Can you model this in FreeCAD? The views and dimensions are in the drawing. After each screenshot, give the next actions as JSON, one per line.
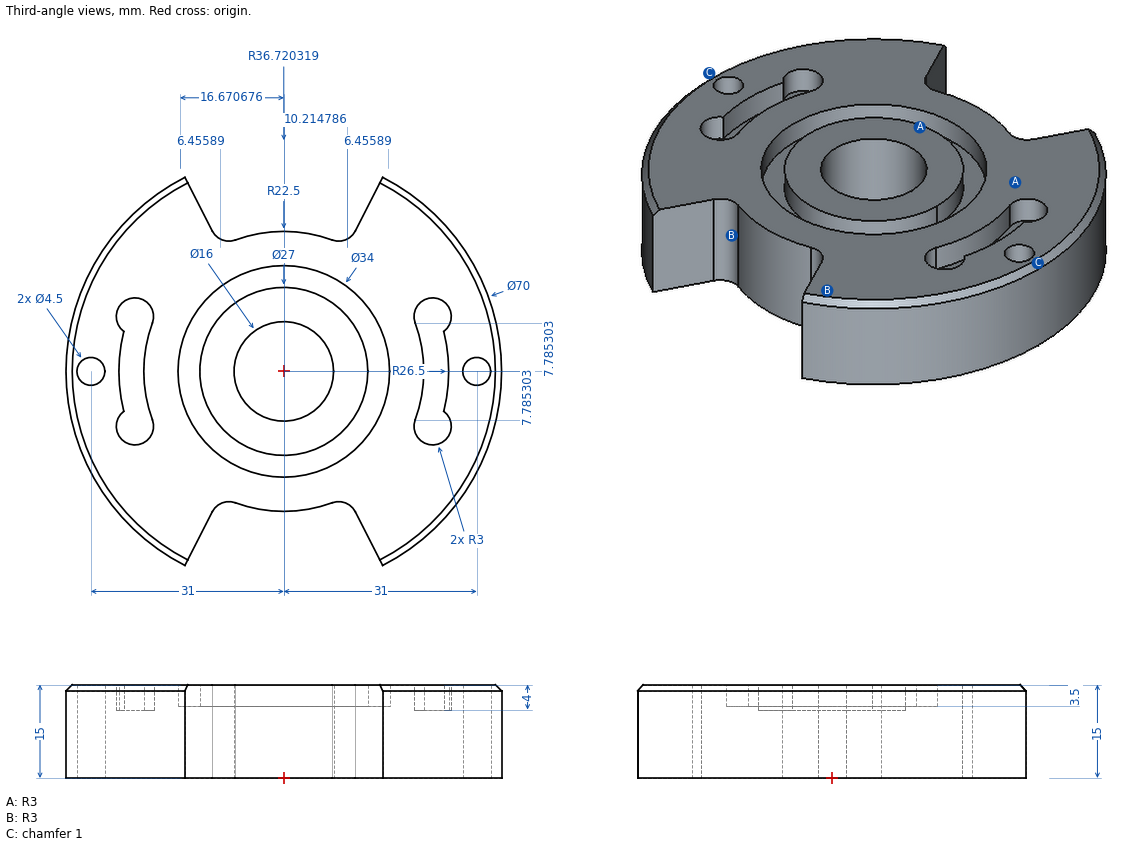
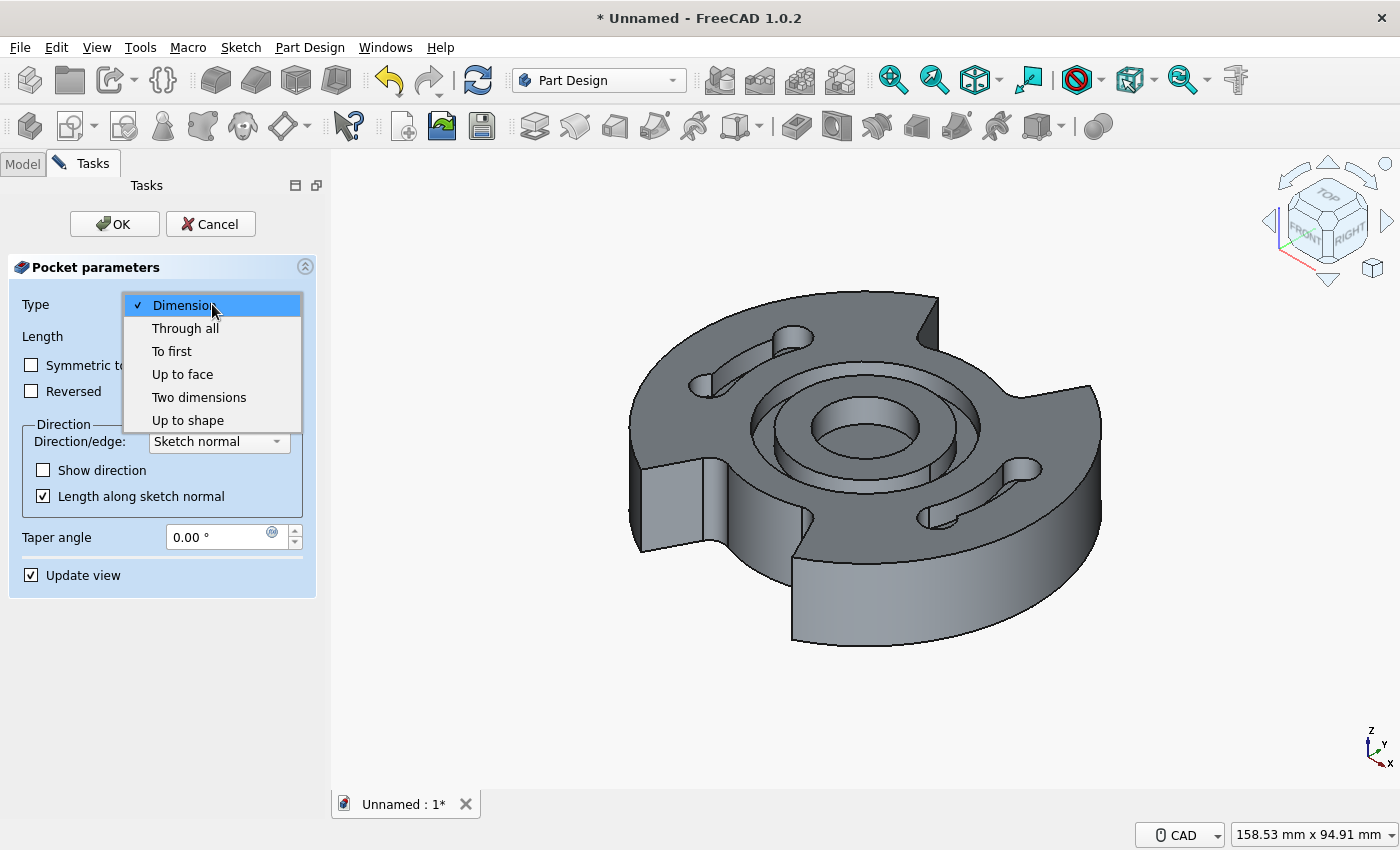
{"action": "left_click", "coordinate": [212, 328]}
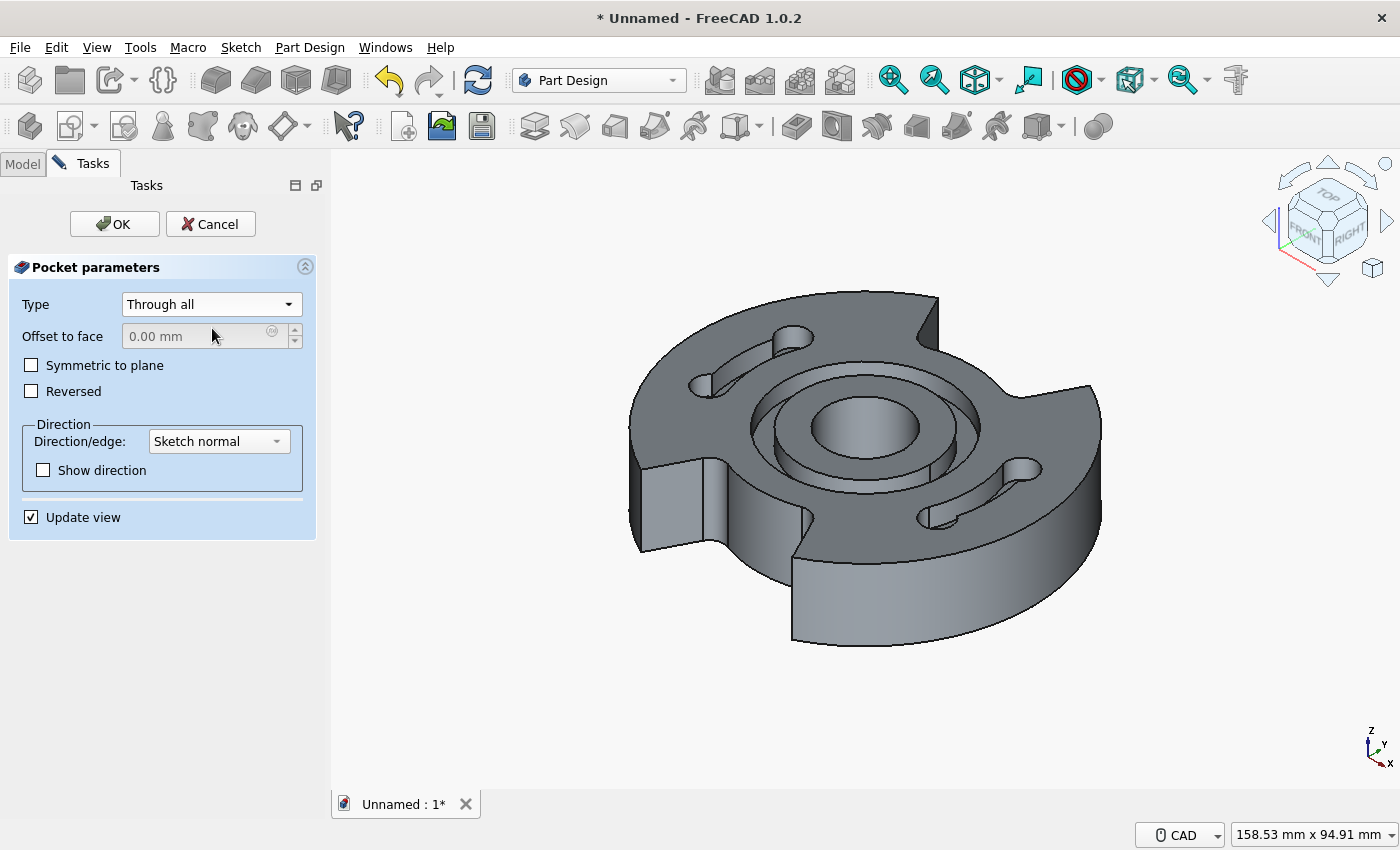
{"action": "left_click", "coordinate": [115, 224]}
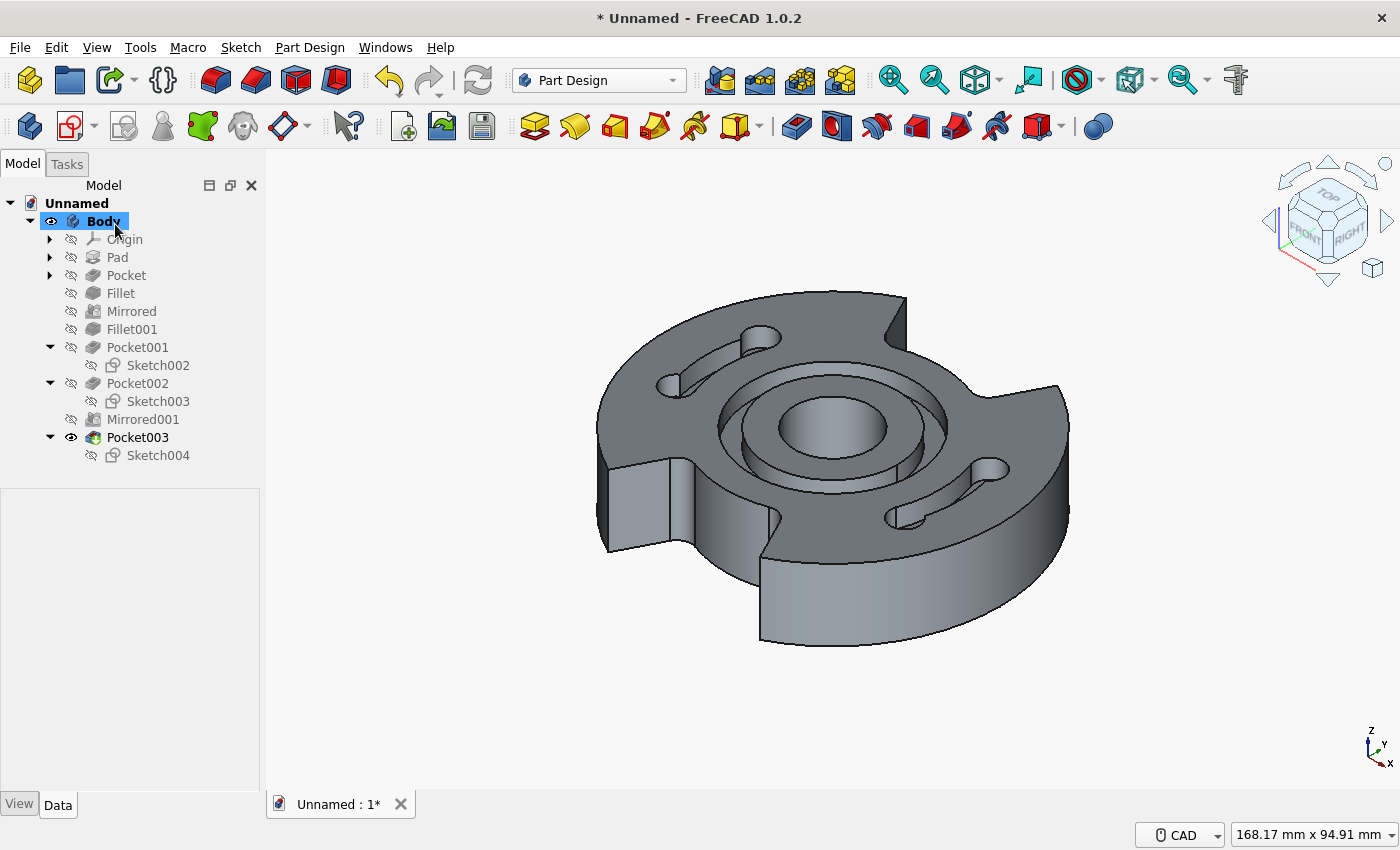
{"action": "left_click", "coordinate": [1013, 433]}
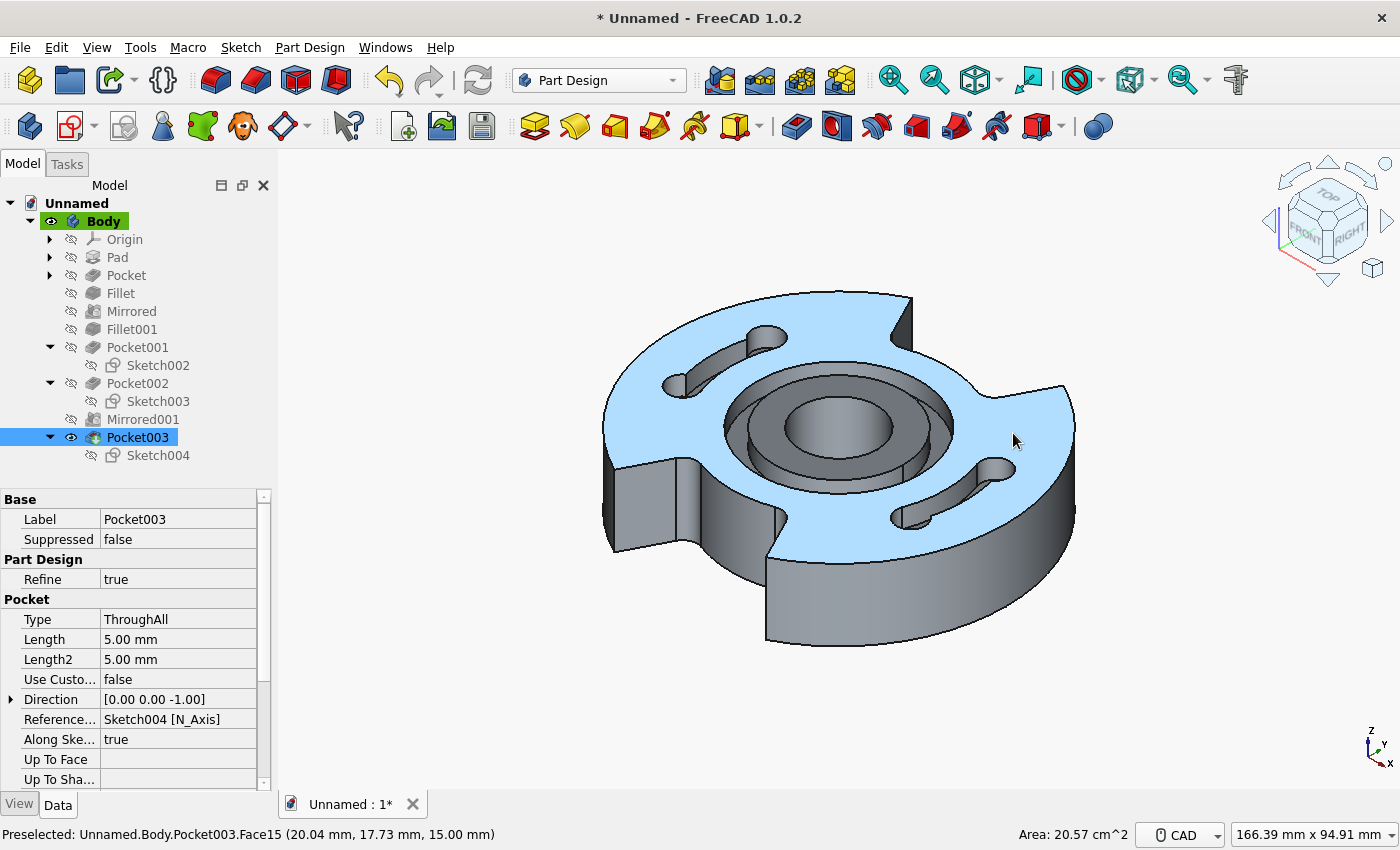
{"action": "left_click", "coordinate": [70, 126]}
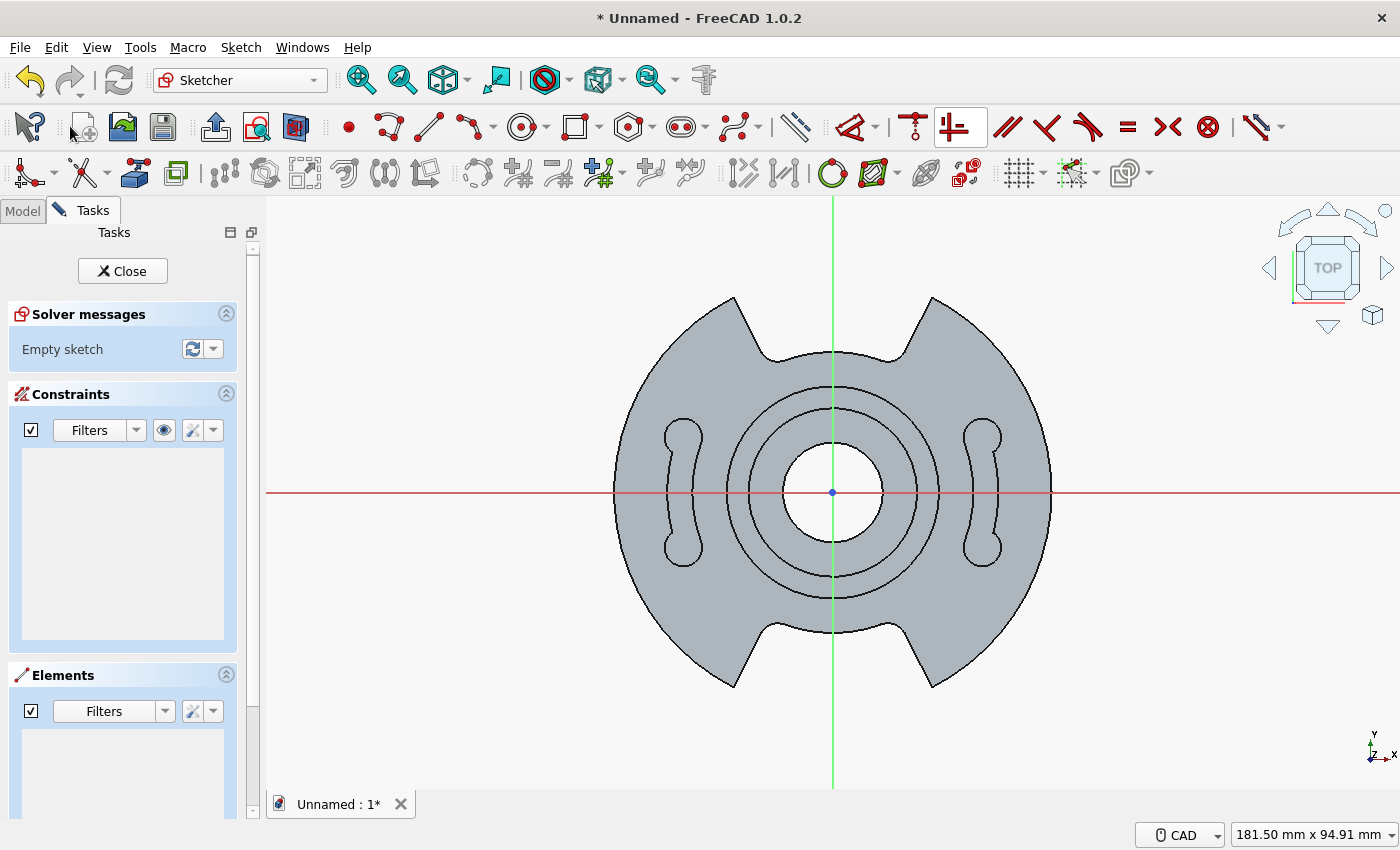
{"action": "scroll", "coordinate": [972, 493], "scroll_direction": "up", "scroll_amount": 2}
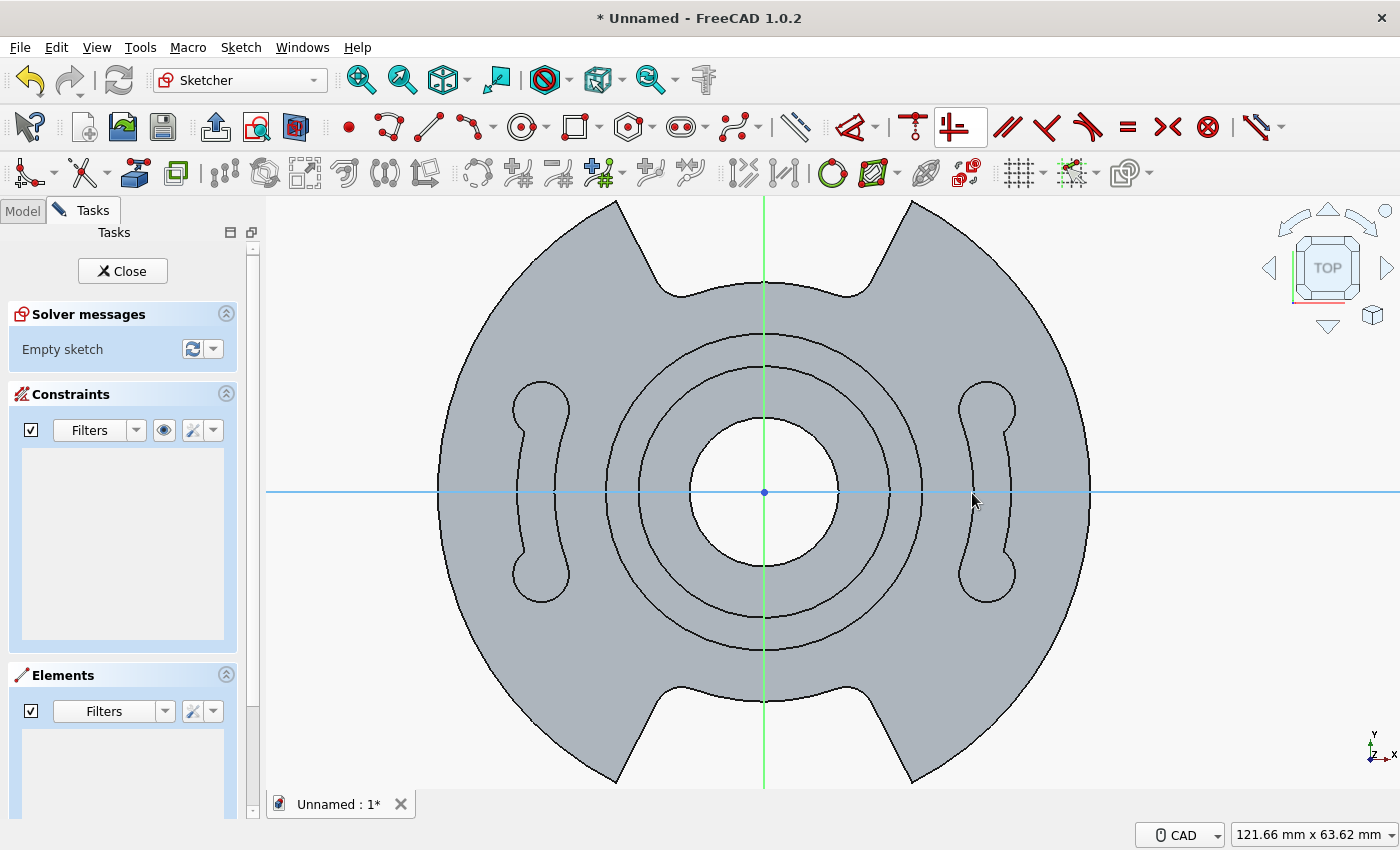
{"action": "left_click", "coordinate": [522, 128]}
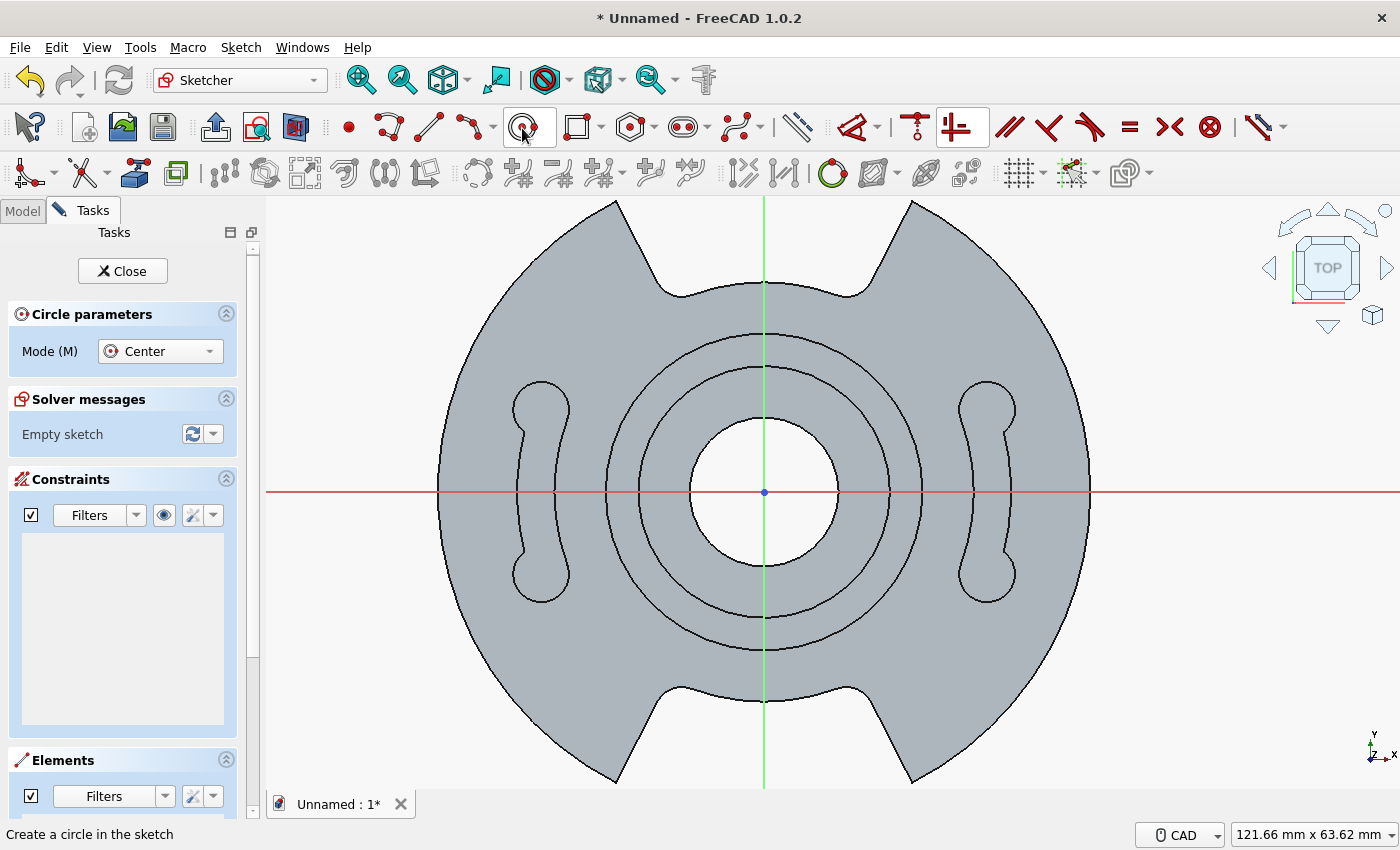
{"action": "left_click", "coordinate": [475, 492]}
{"action": "mouse_move", "coordinate": [490, 477]}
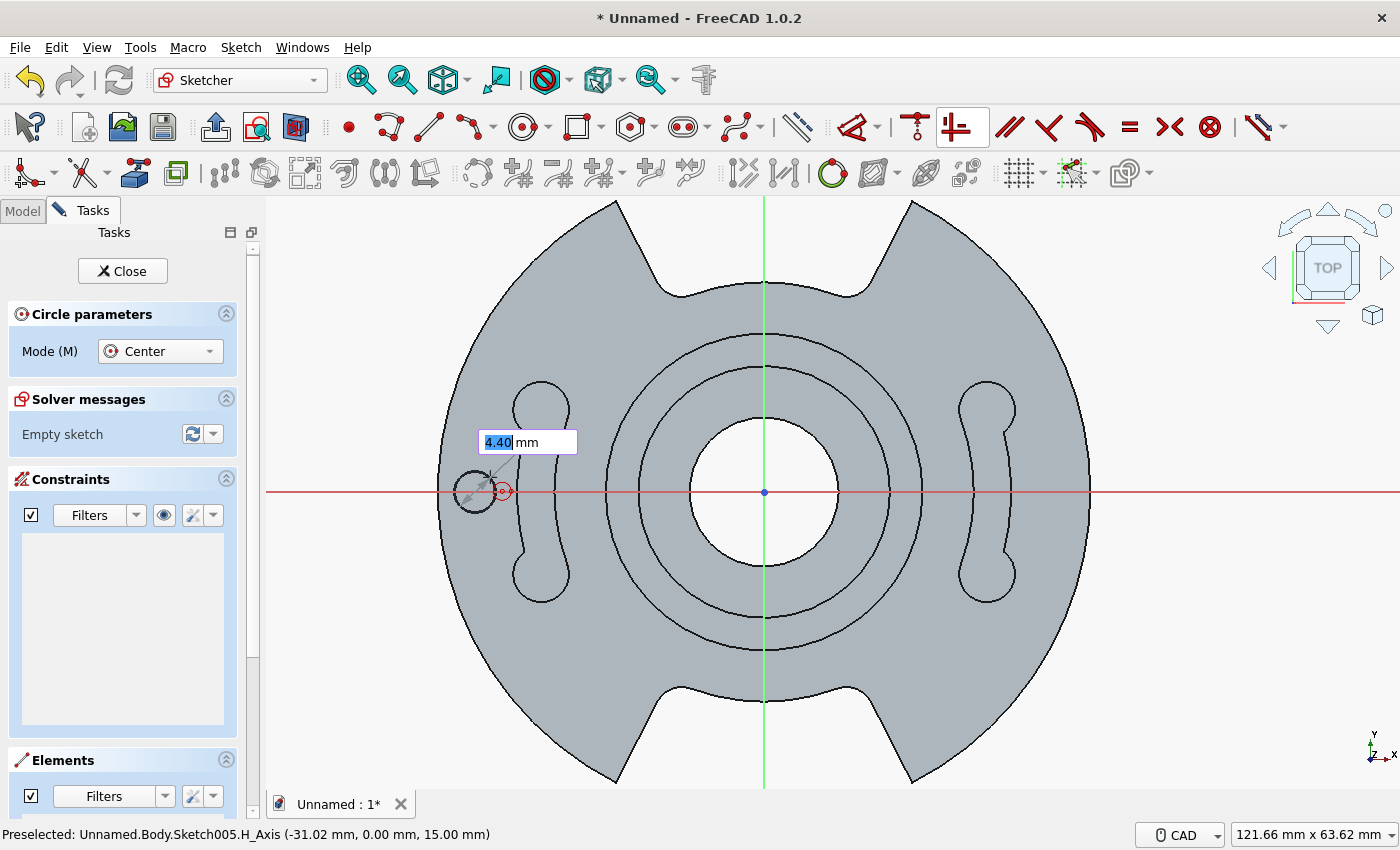
{"action": "type", "text": "4.5"}
{"action": "key", "text": "Return"}